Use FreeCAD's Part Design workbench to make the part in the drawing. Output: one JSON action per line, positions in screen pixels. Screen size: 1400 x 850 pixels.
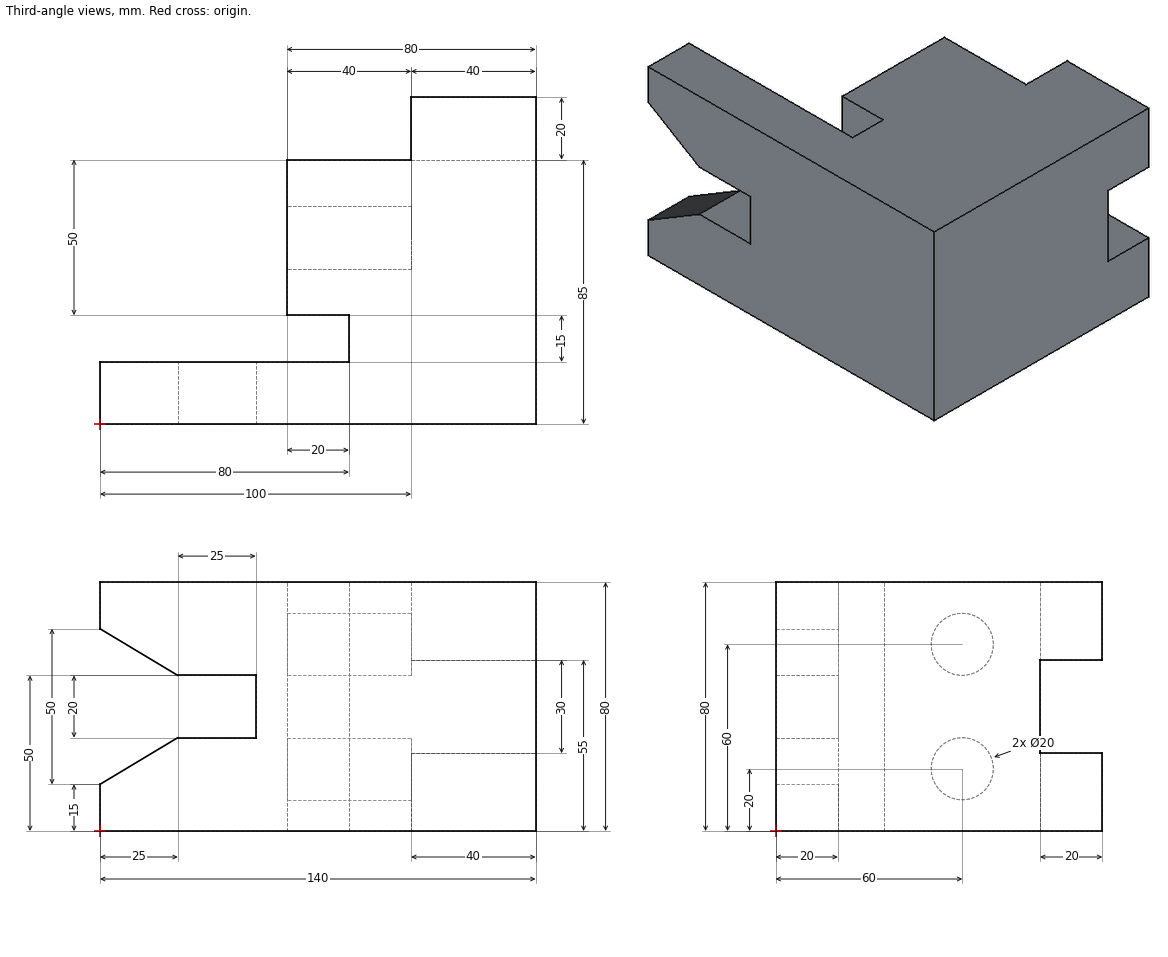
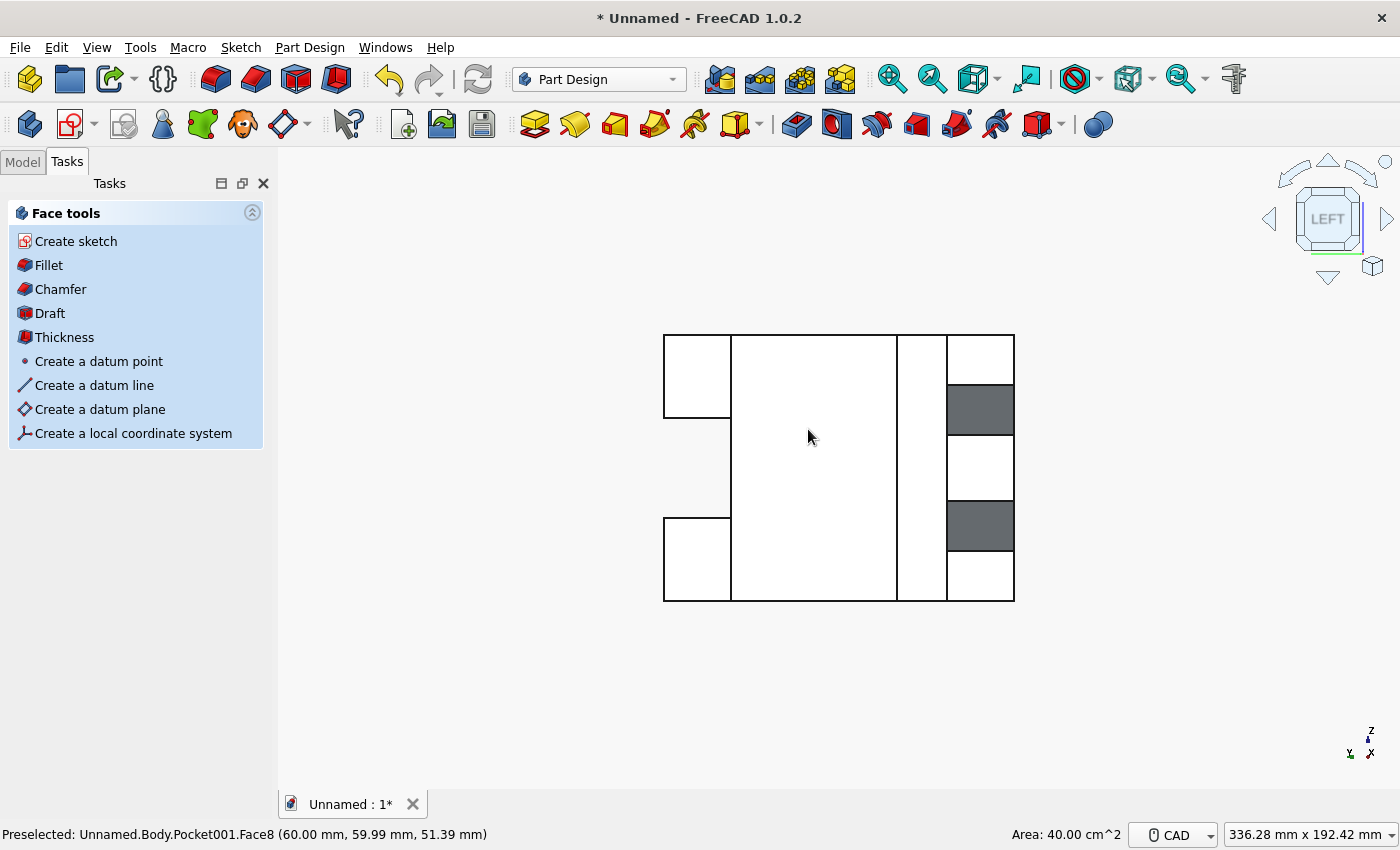
{"action": "left_click", "coordinate": [70, 124]}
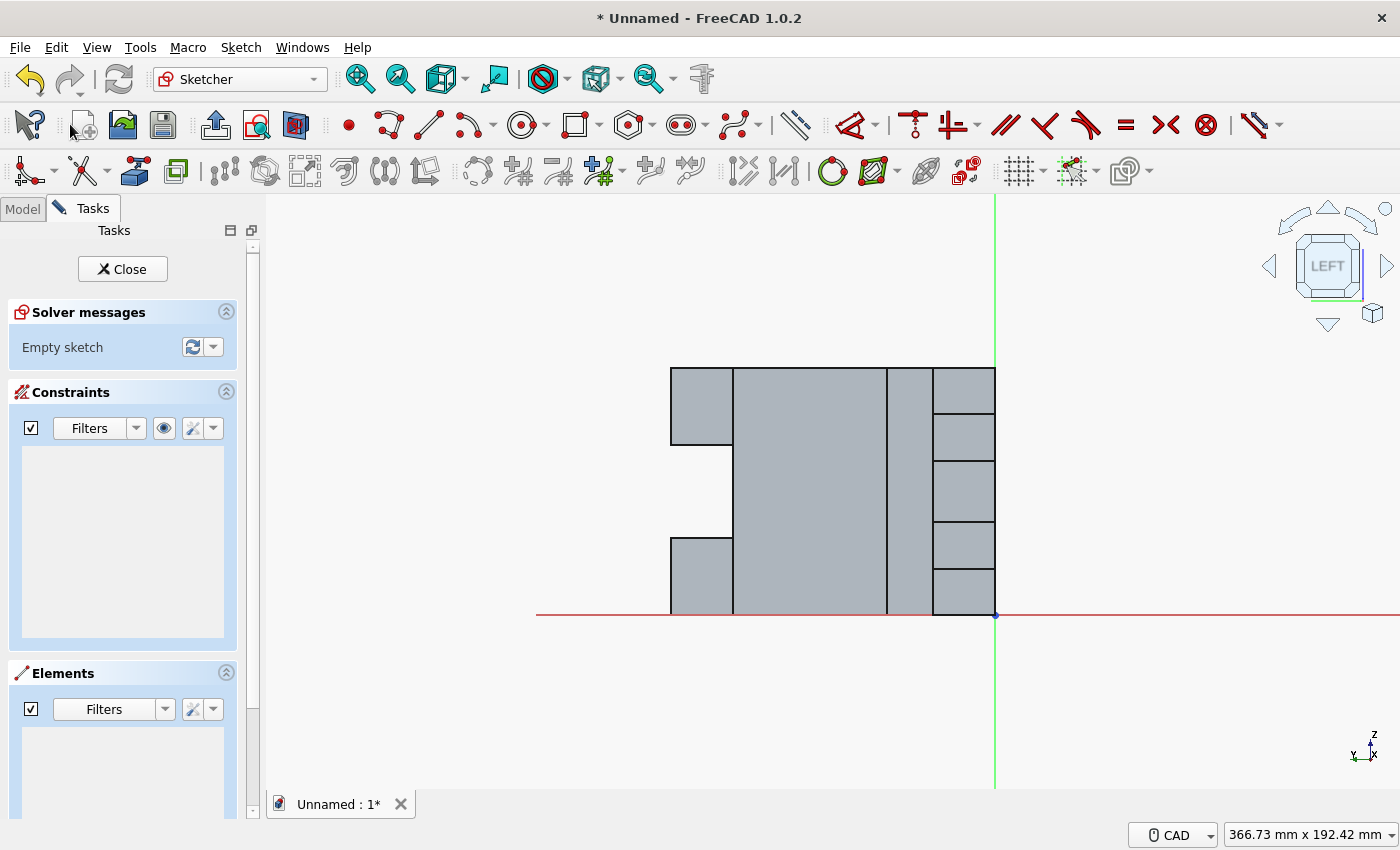
{"action": "scroll", "coordinate": [1036, 526], "scroll_direction": "up", "scroll_amount": 3}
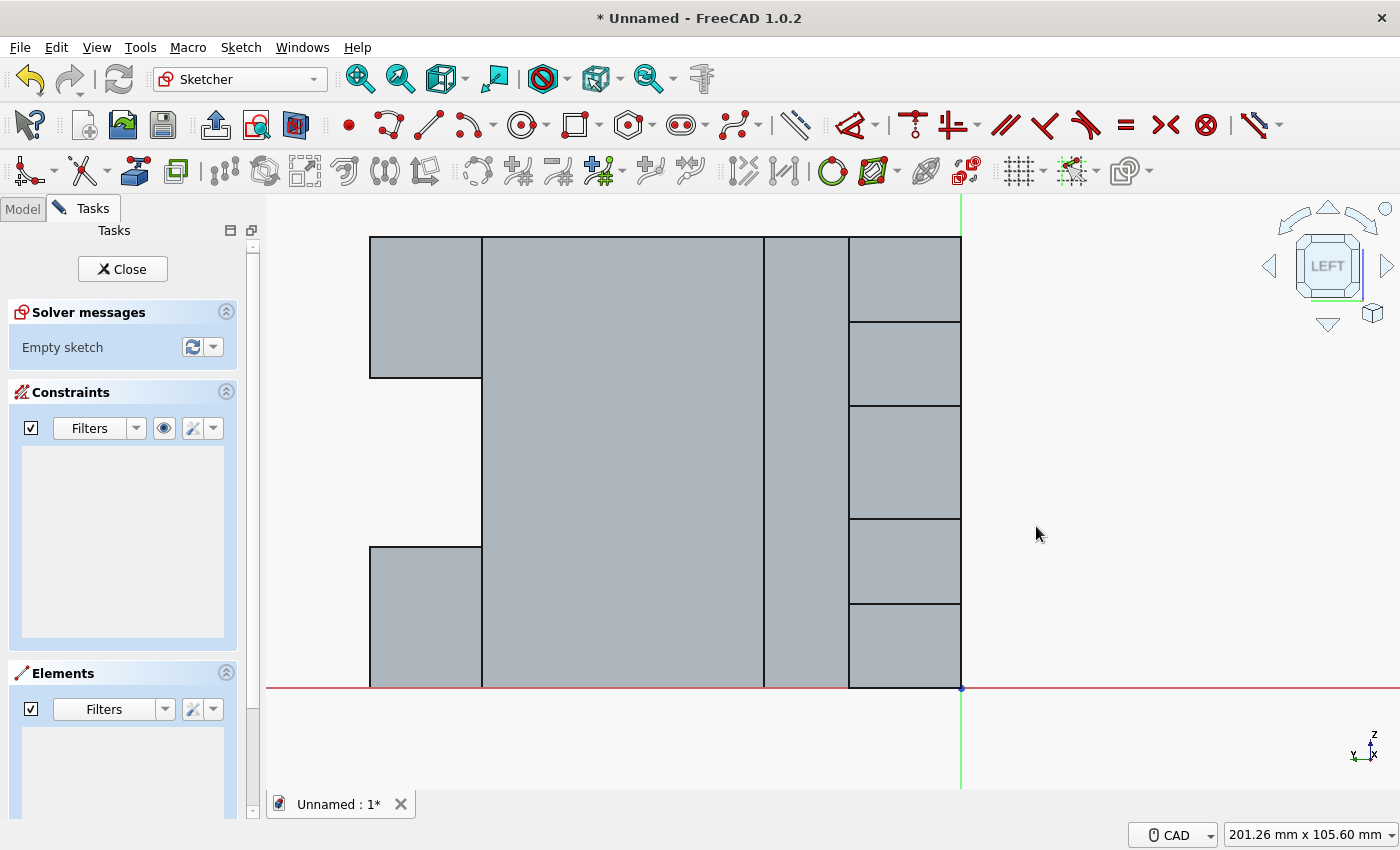
{"action": "key", "text": "g c"}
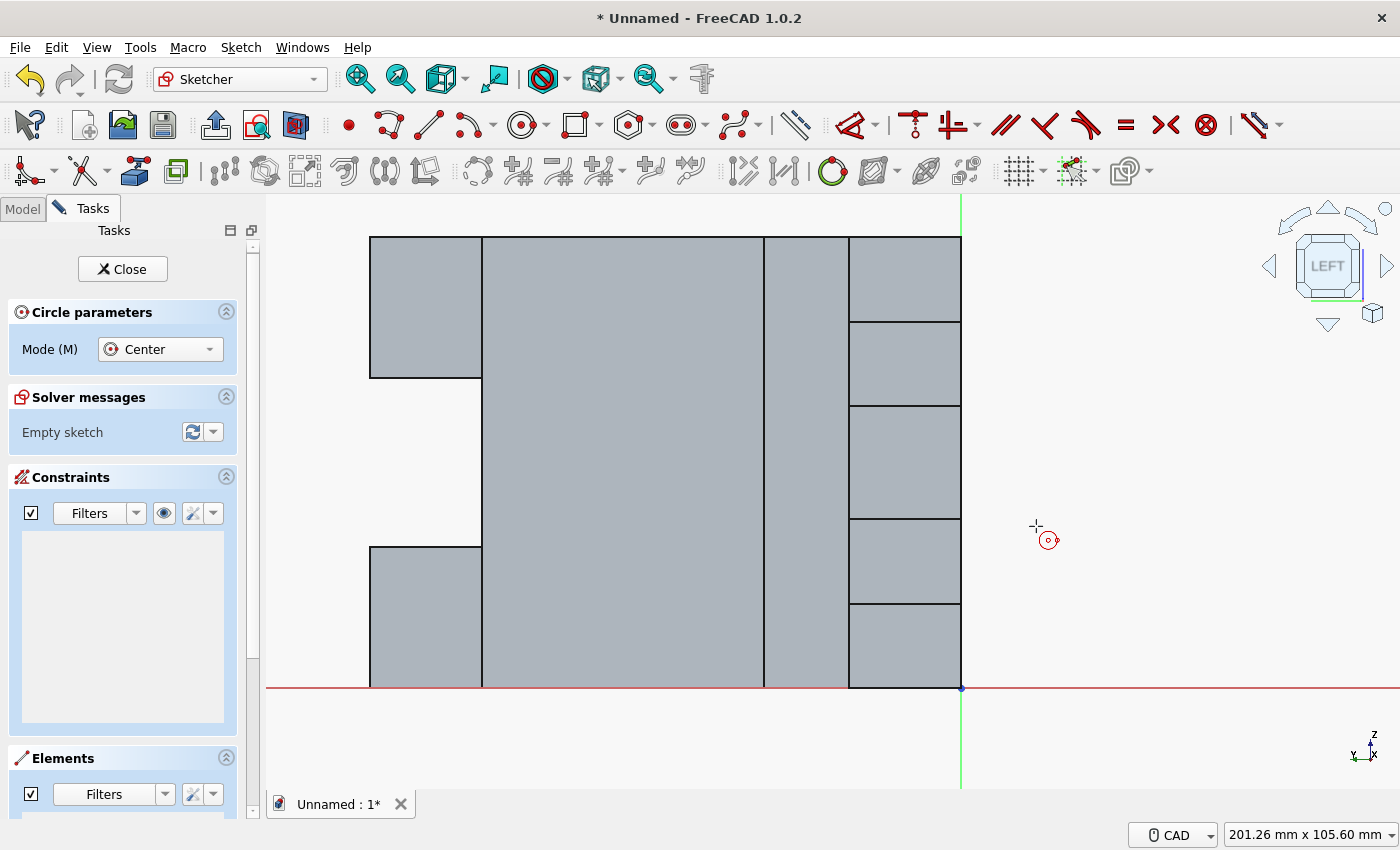
{"action": "left_click", "coordinate": [623, 575]}
{"action": "mouse_move", "coordinate": [663, 536]}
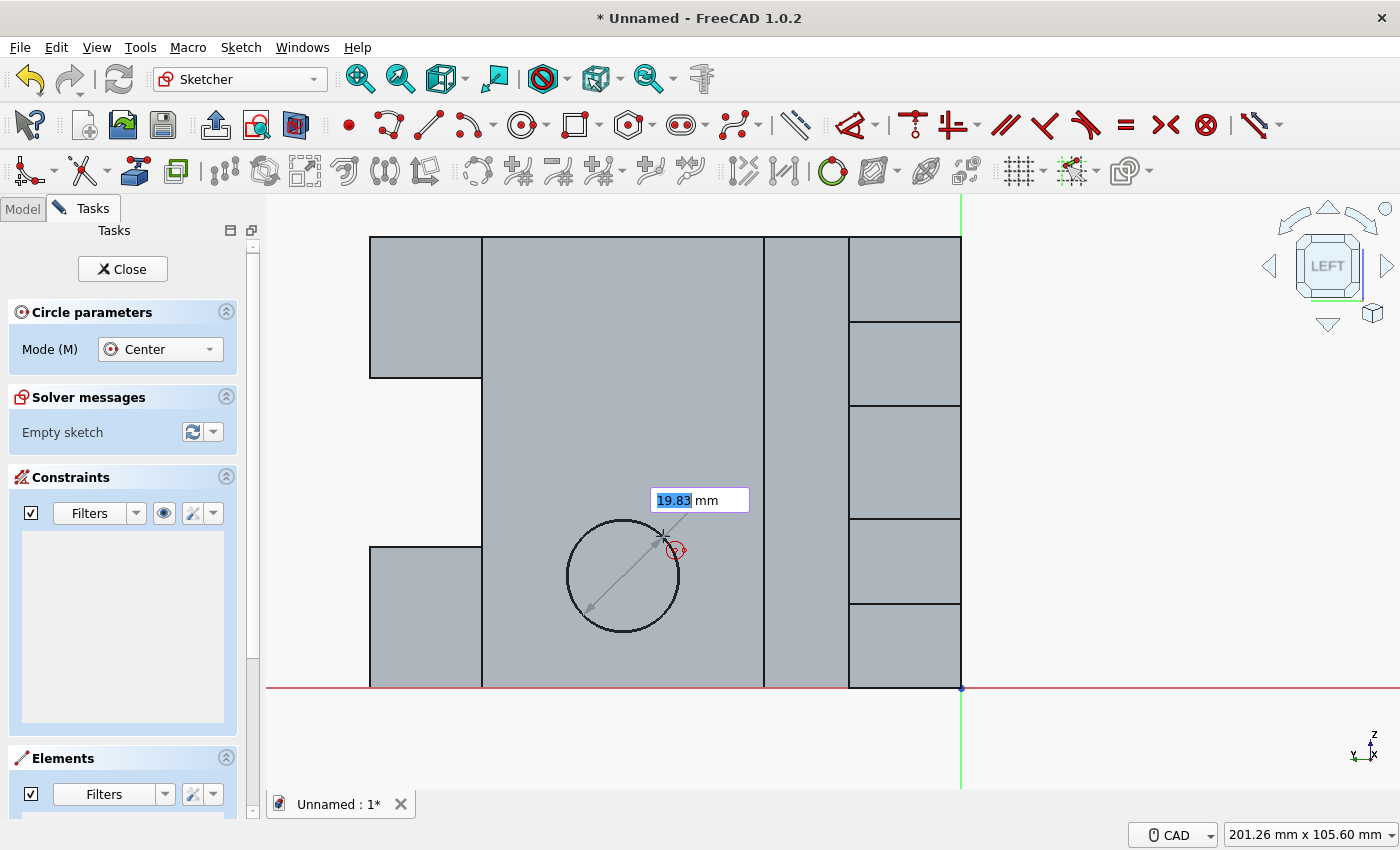
{"action": "type", "text": "20"}
{"action": "key", "text": "Return"}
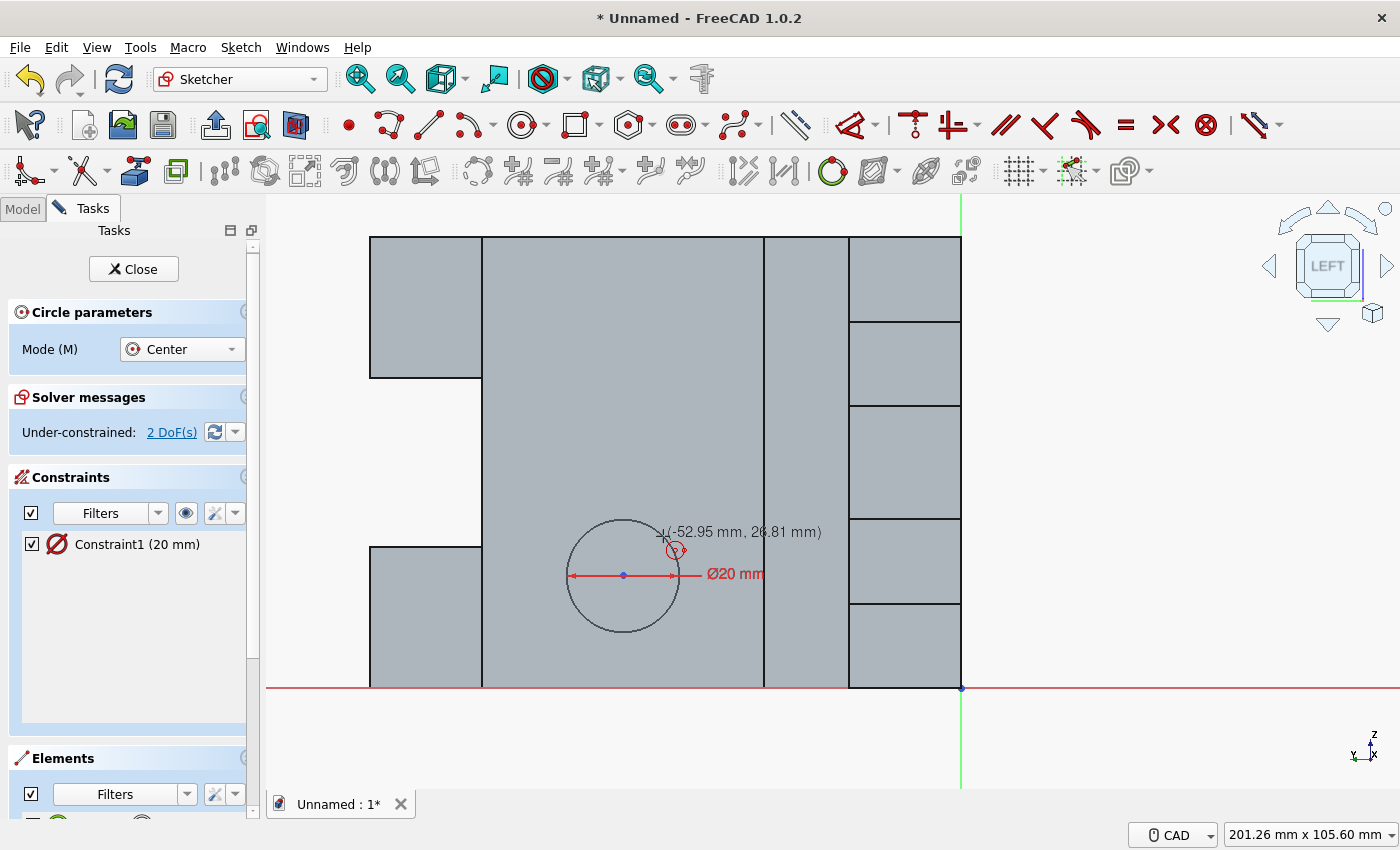
{"action": "left_click", "coordinate": [623, 350]}
{"action": "mouse_move", "coordinate": [663, 310]}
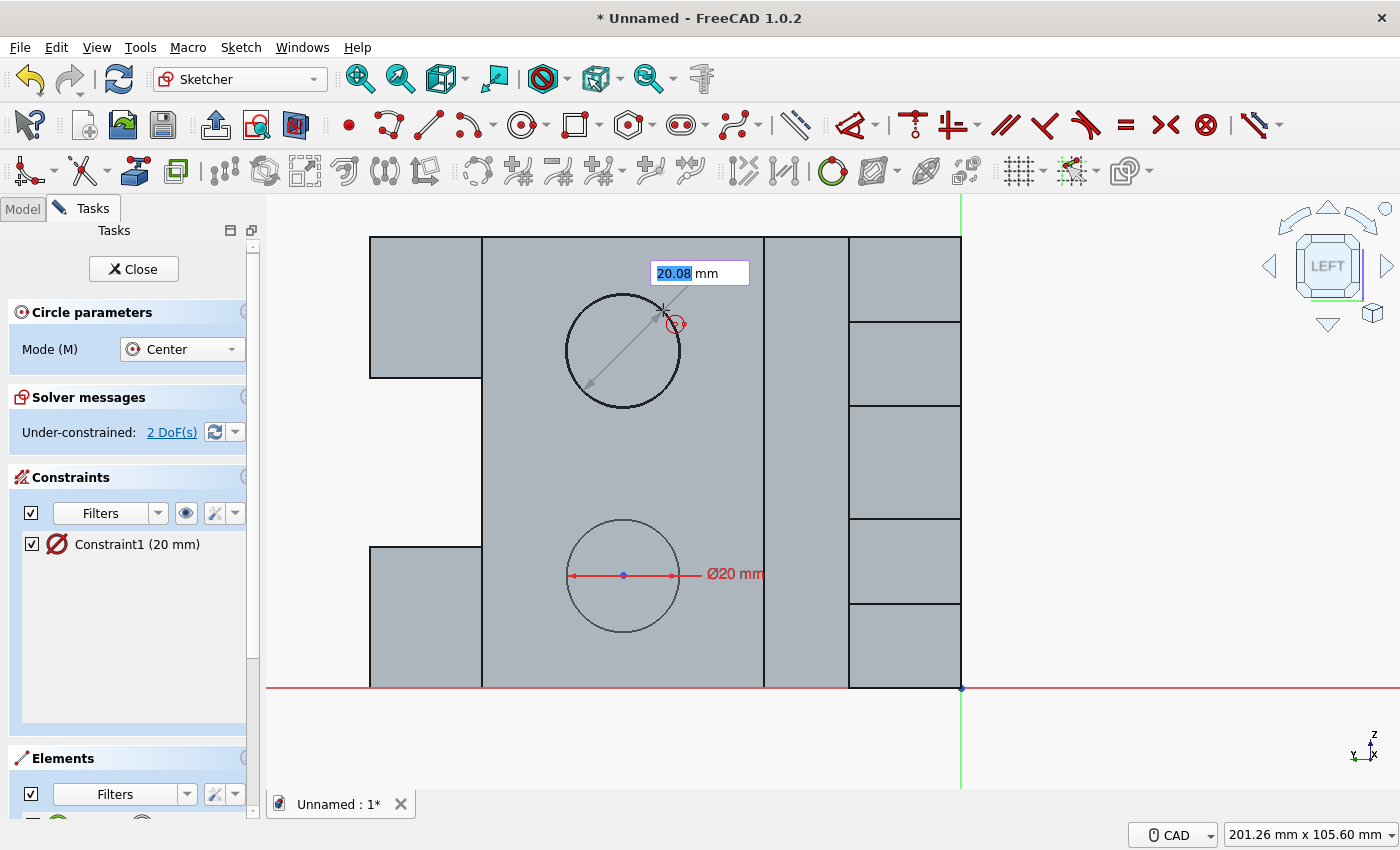
{"action": "type", "text": "20"}
{"action": "key", "text": "Return"}
{"action": "key", "text": "Escape"}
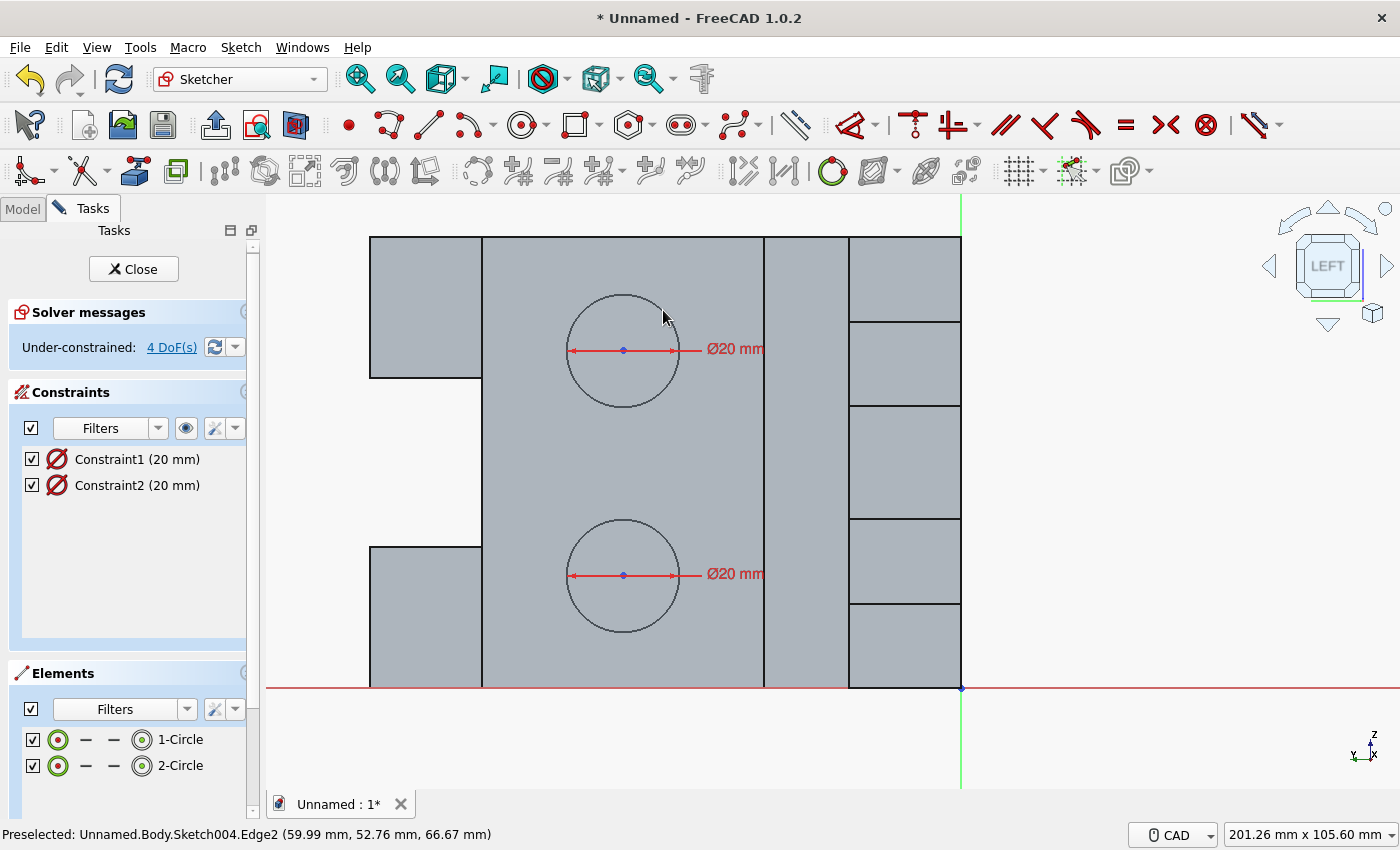
{"action": "left_click", "coordinate": [623, 576]}